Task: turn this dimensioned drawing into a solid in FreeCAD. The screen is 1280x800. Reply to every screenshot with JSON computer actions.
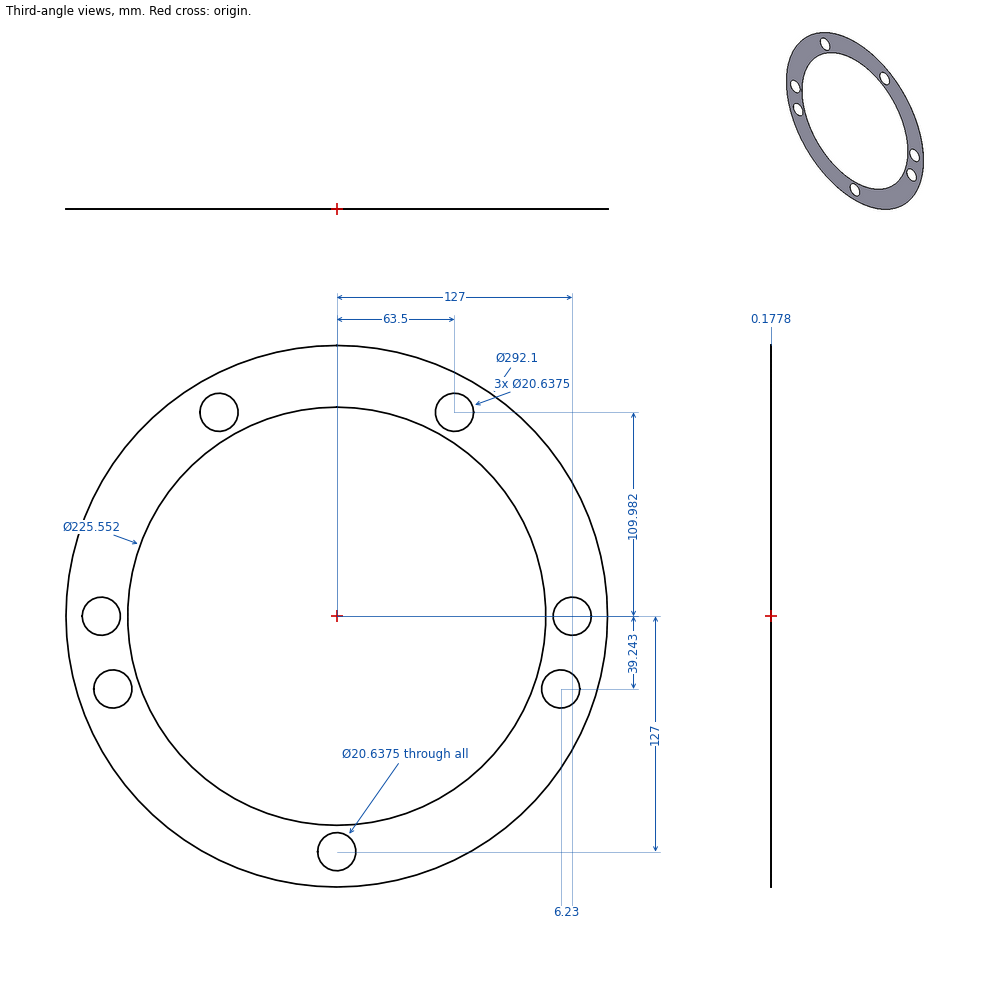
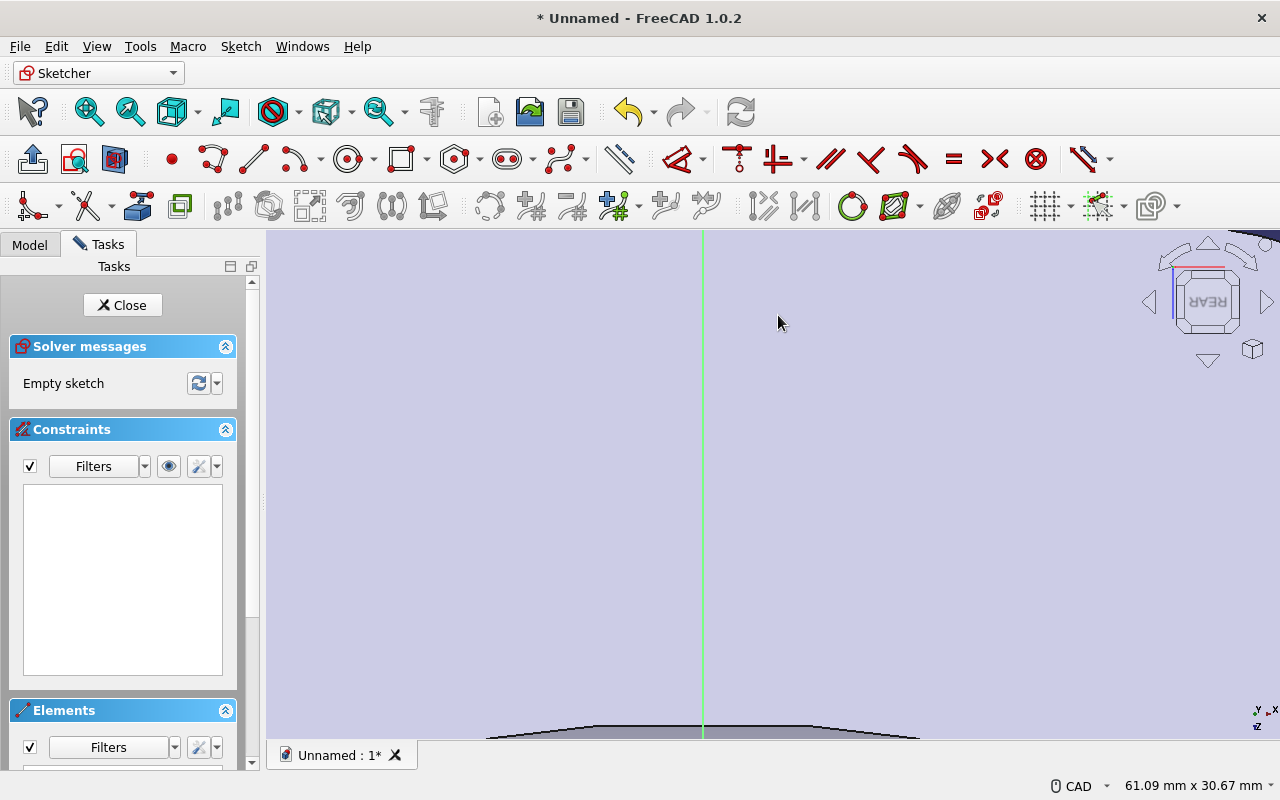
{"action": "left_click", "coordinate": [348, 160]}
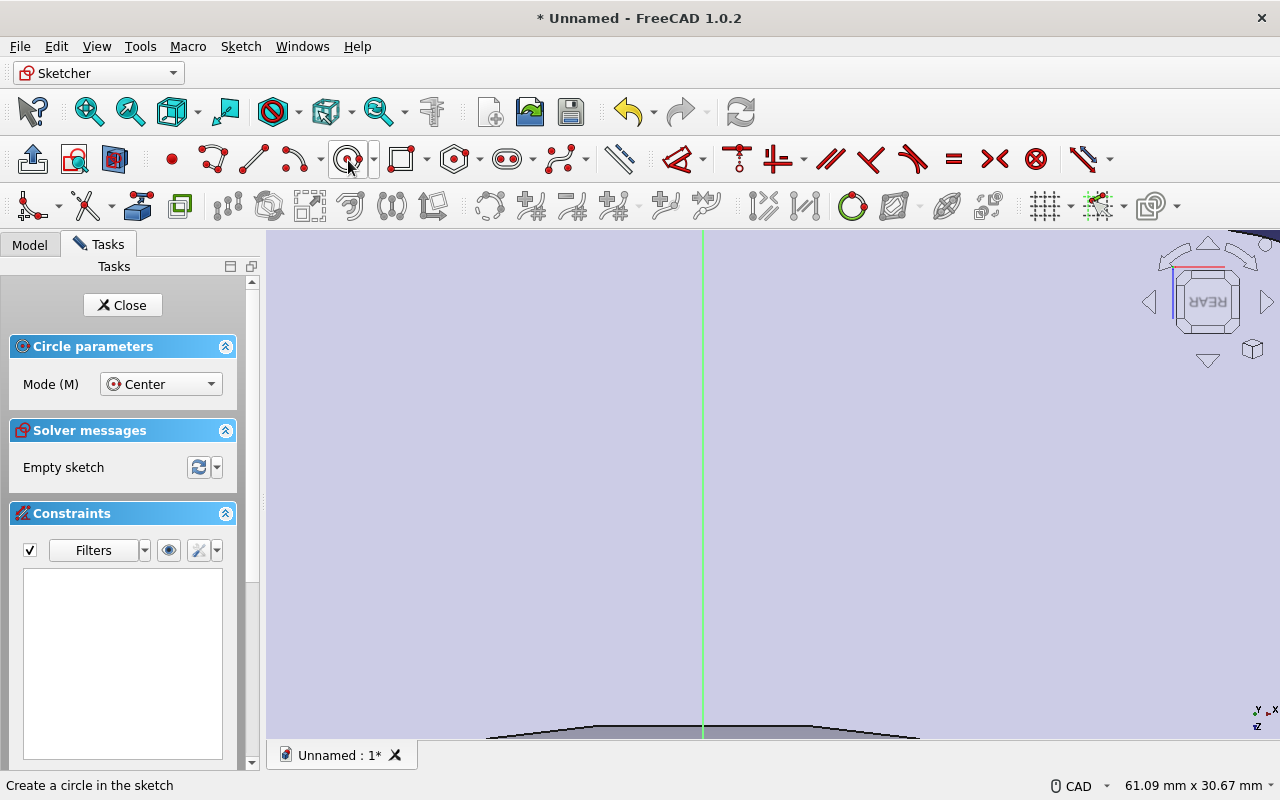
{"action": "left_click", "coordinate": [703, 487]}
{"action": "mouse_move", "coordinate": [824, 366]}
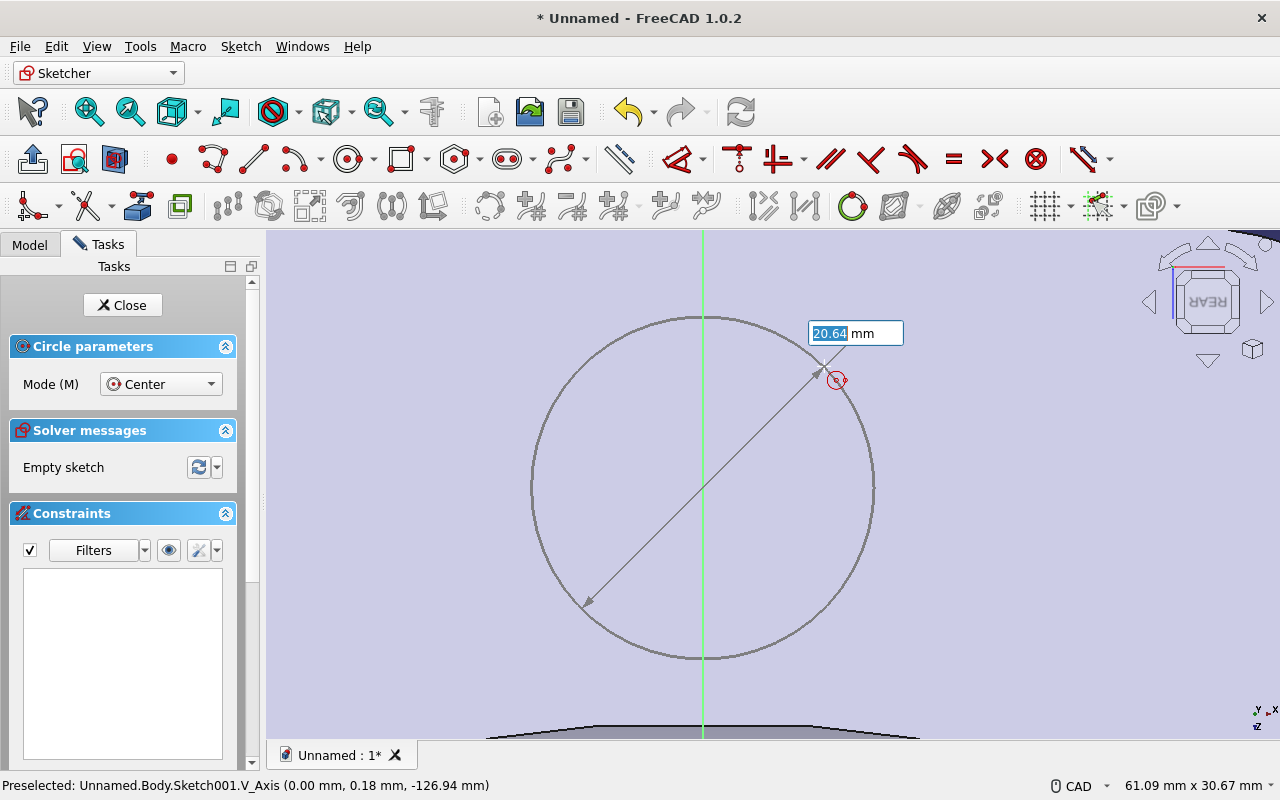
{"action": "type", "text": "20.6375"}
{"action": "key", "text": "Return"}
{"action": "key", "text": "Escape"}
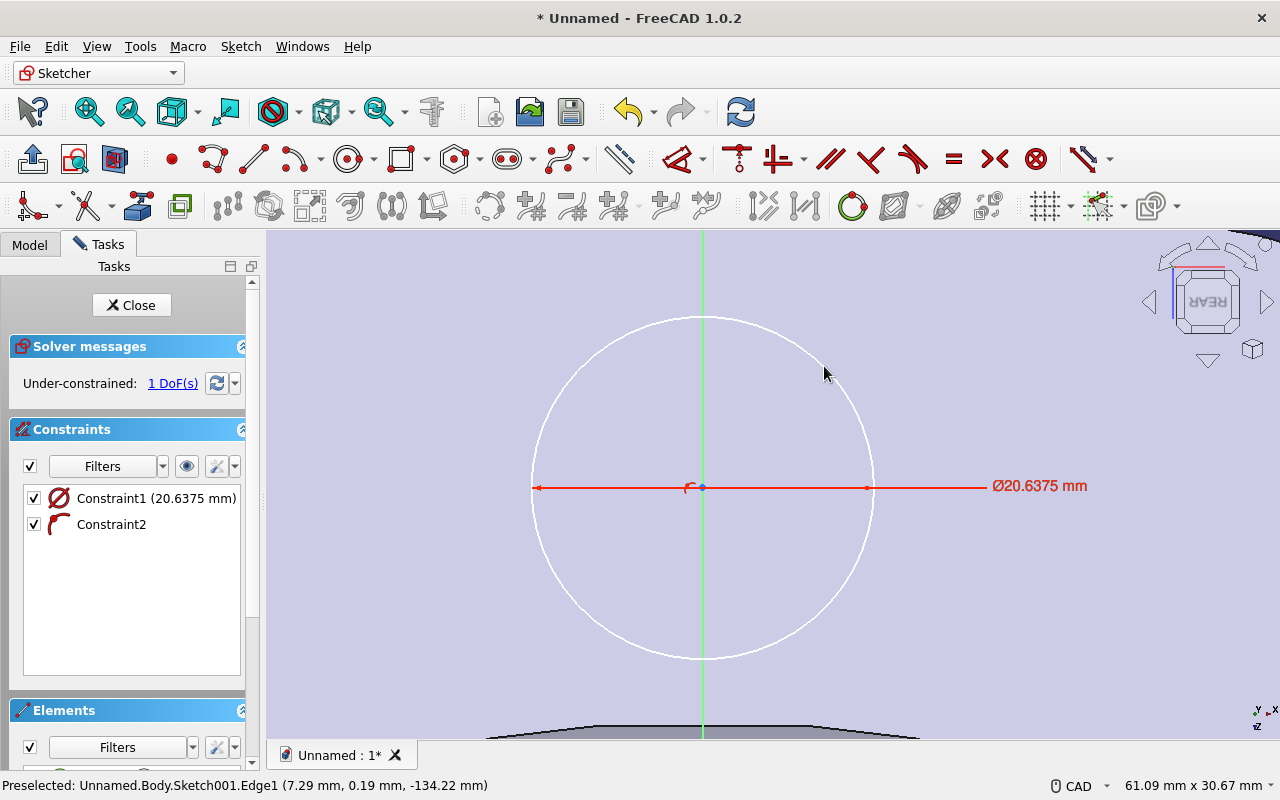
{"action": "key", "text": "d"}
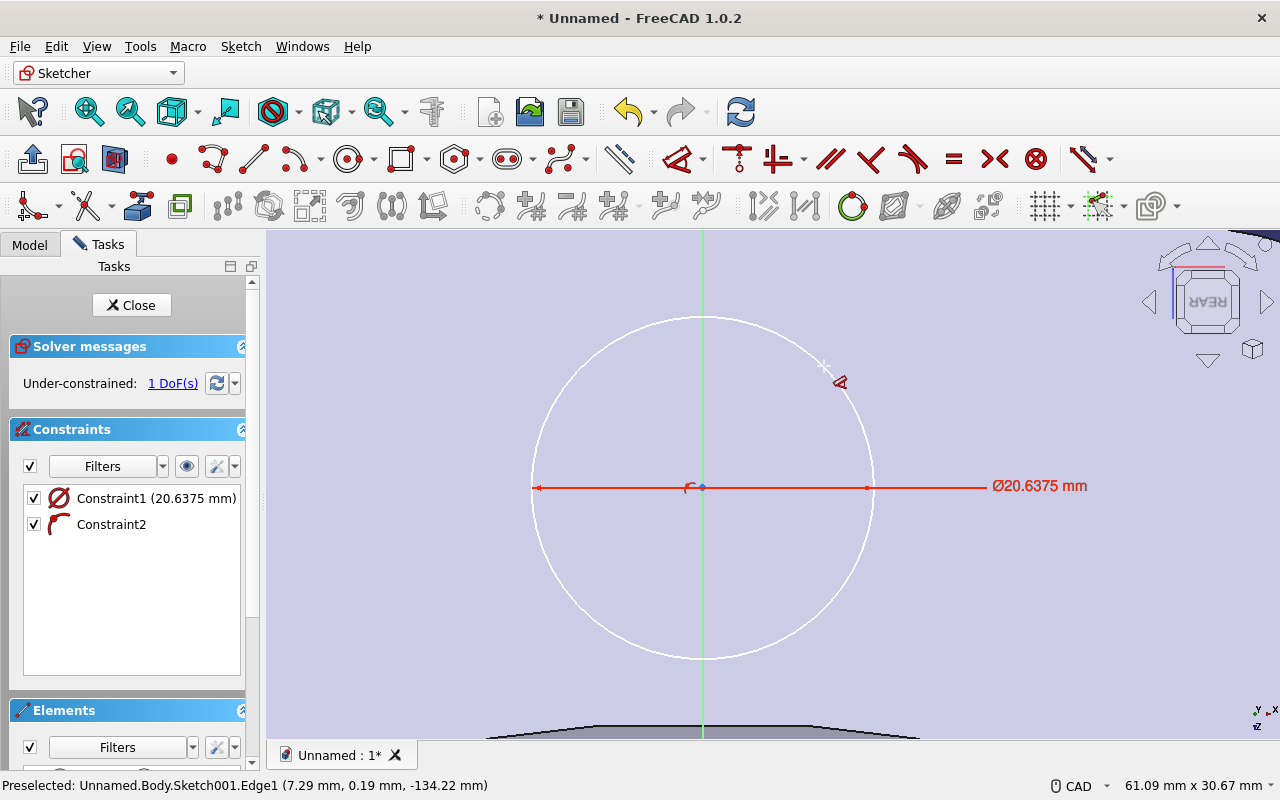
{"action": "left_click", "coordinate": [703, 488]}
{"action": "left_click", "coordinate": [737, 599]}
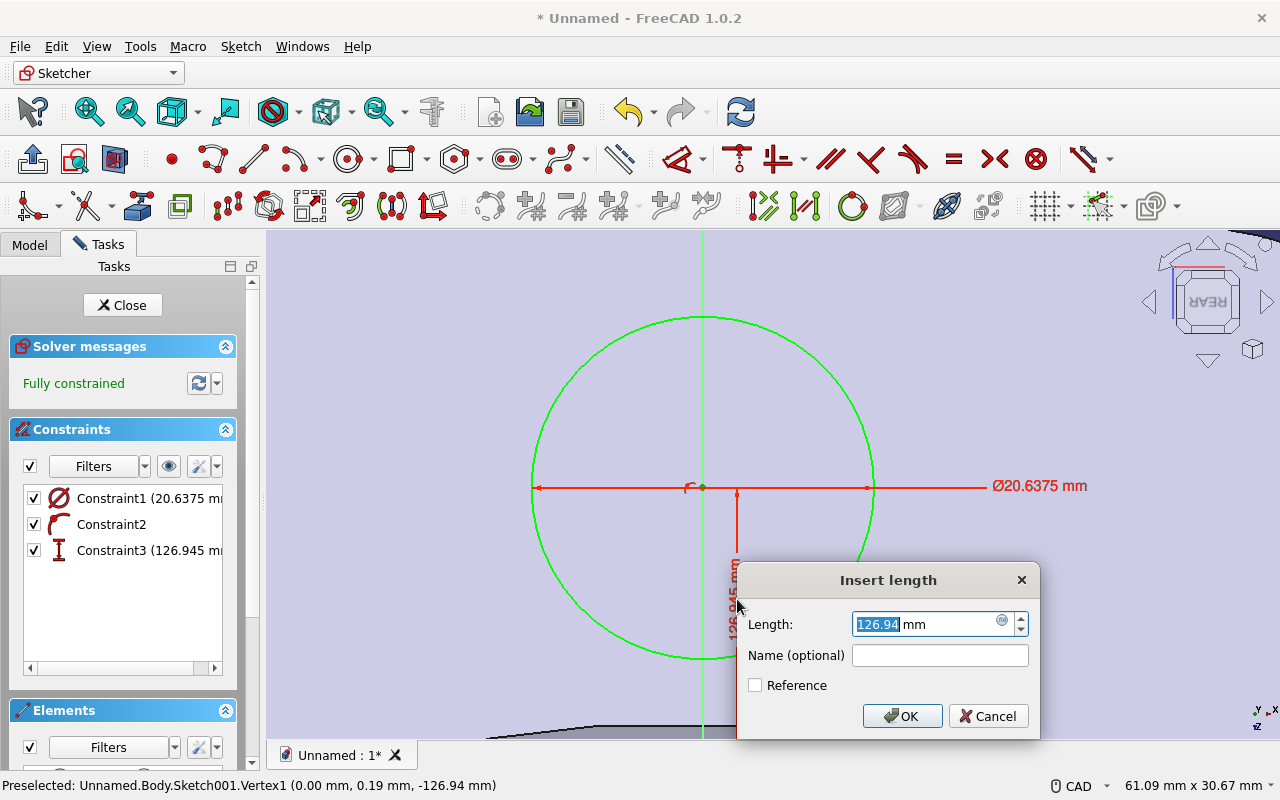
{"action": "type", "text": "127"}
{"action": "key", "text": "Return"}
{"action": "key", "text": "Escape"}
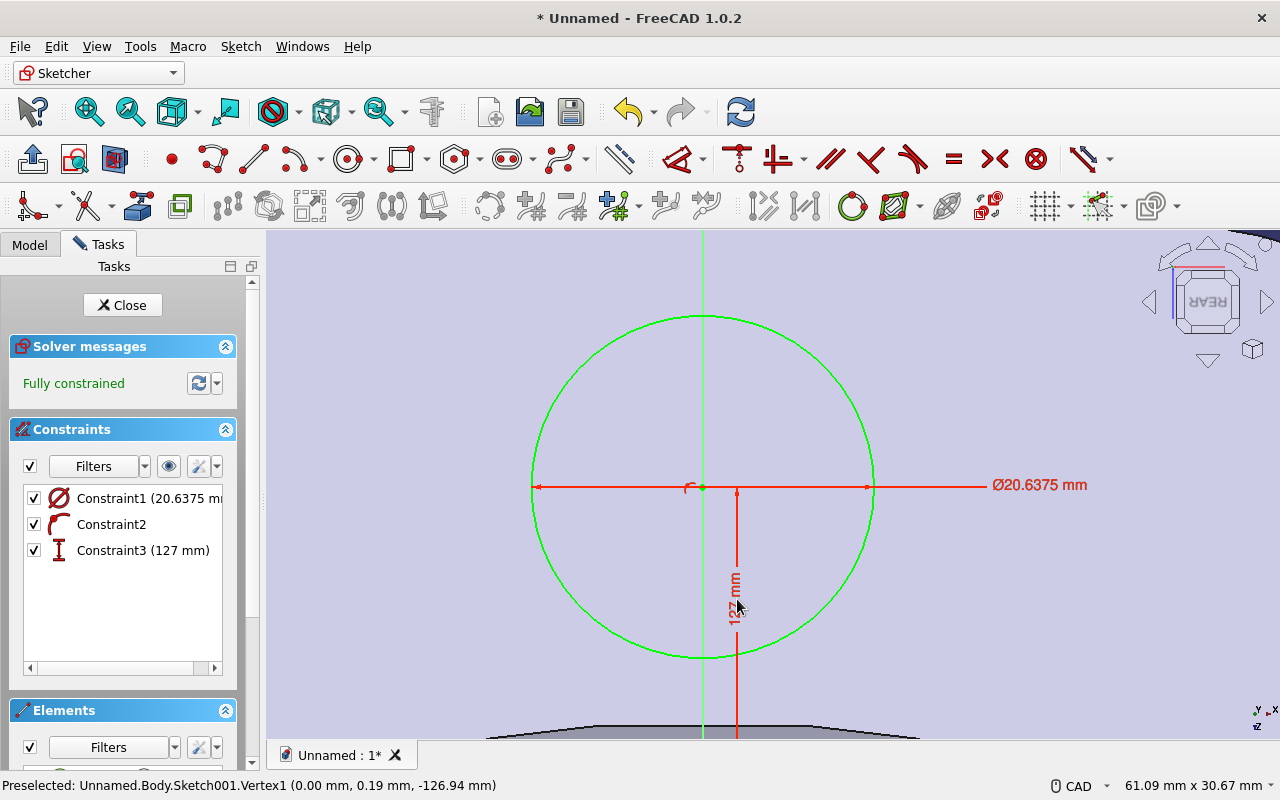
{"action": "left_click", "coordinate": [123, 305]}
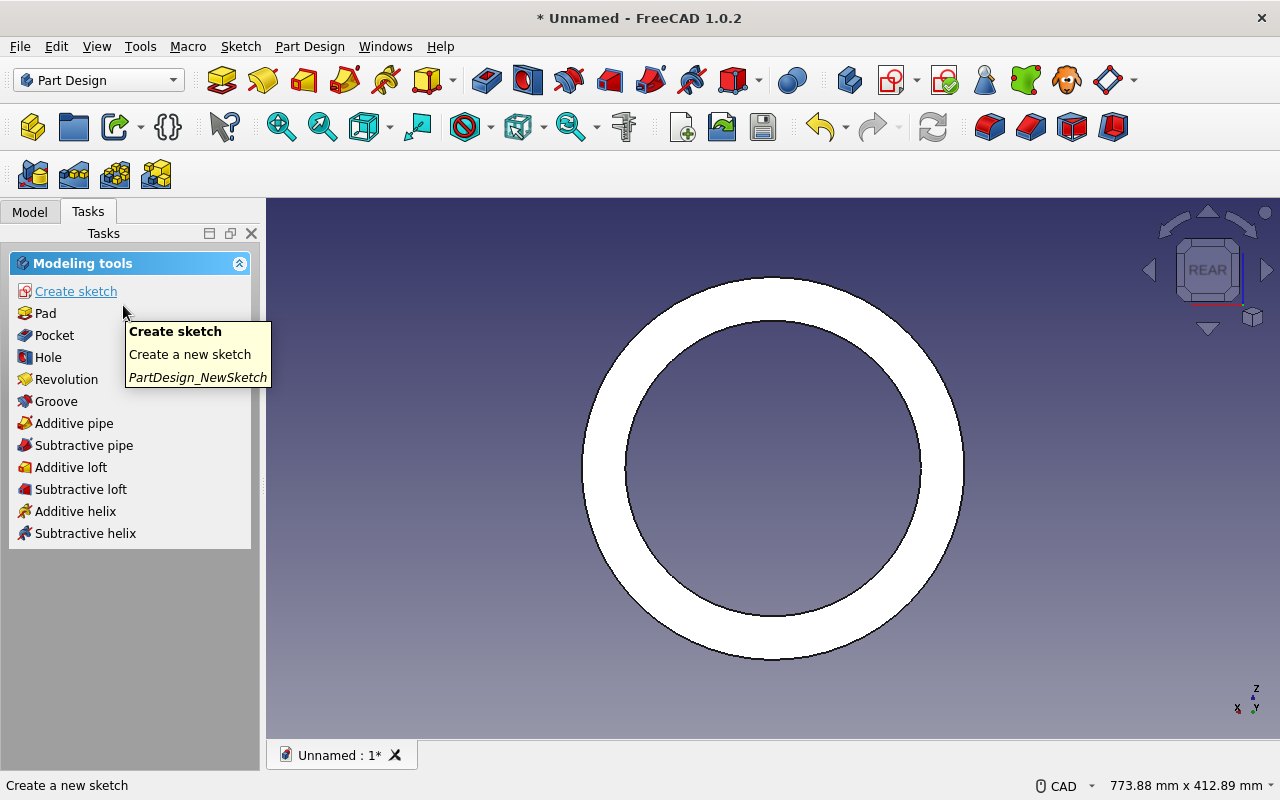
{"action": "left_click", "coordinate": [528, 80]}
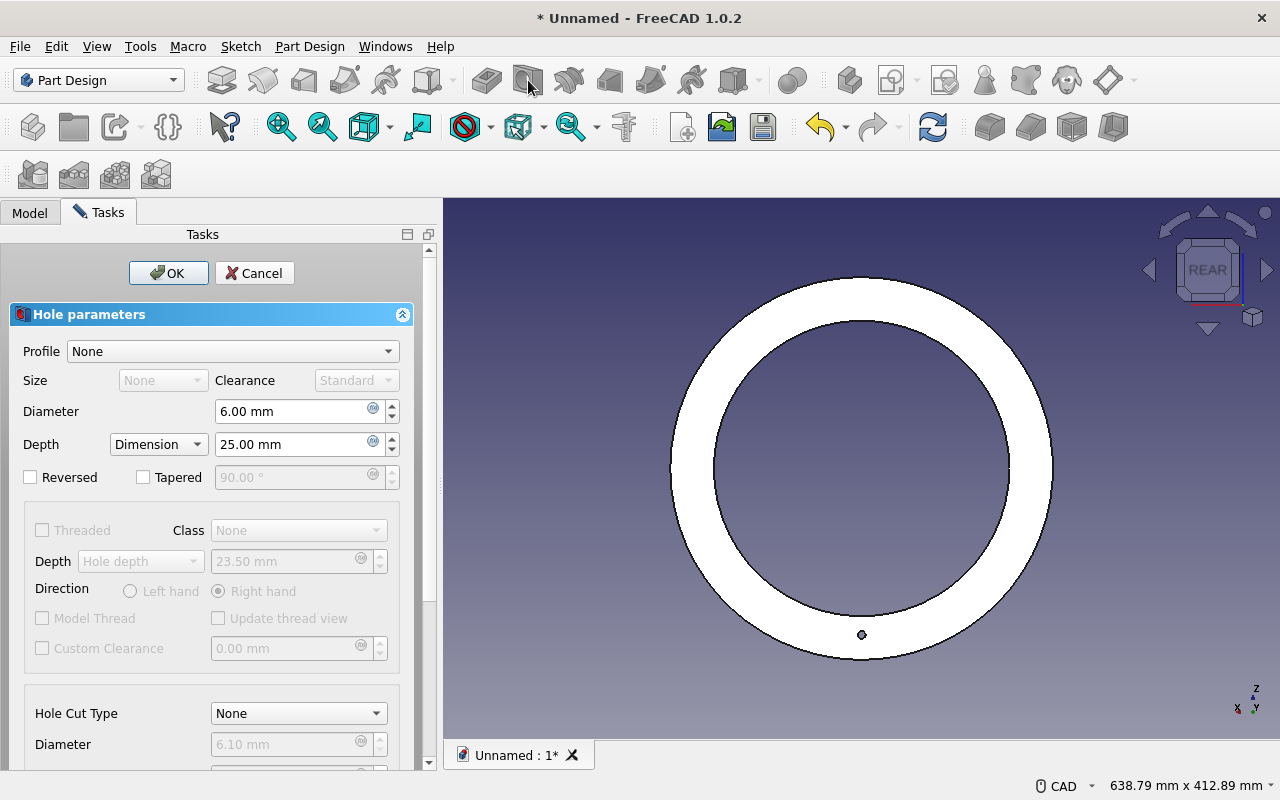
{"action": "triple_click", "coordinate": [300, 412]}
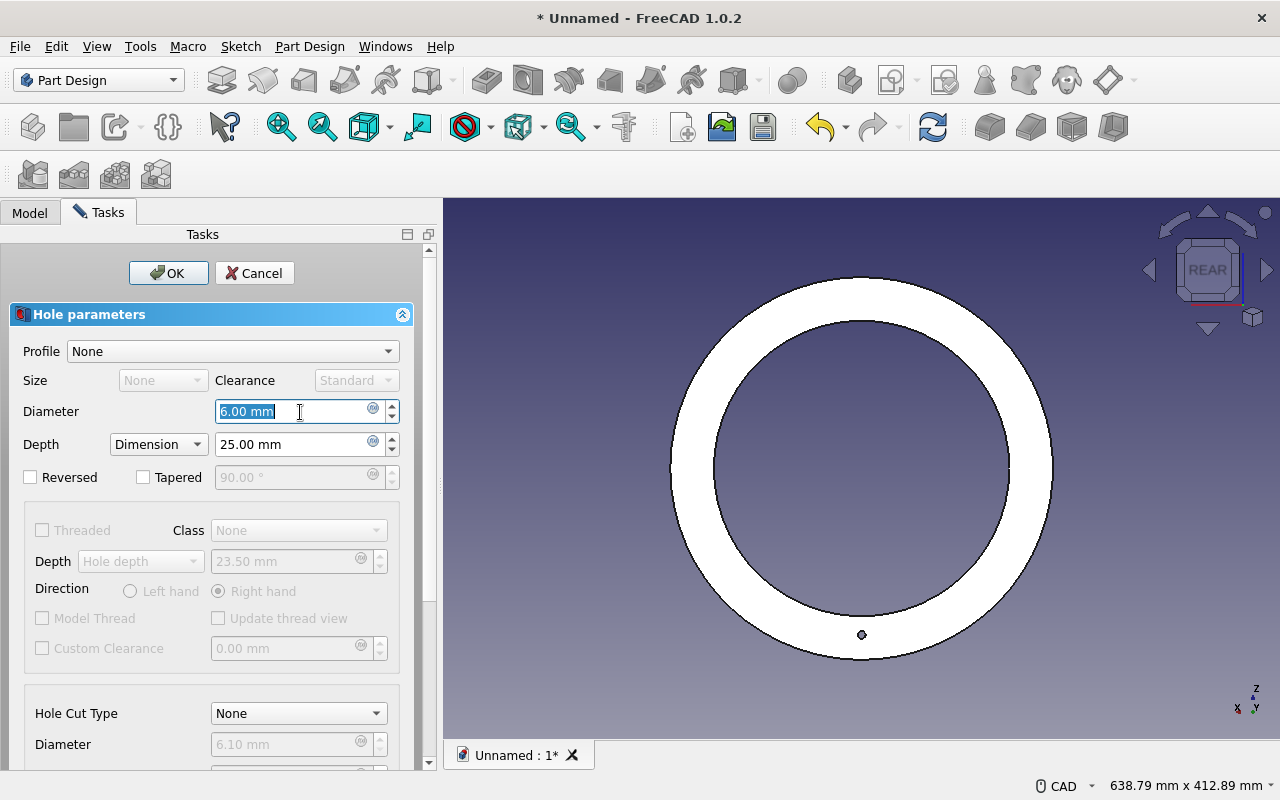
{"action": "type", "text": "20.6375"}
{"action": "key", "text": "Tab"}